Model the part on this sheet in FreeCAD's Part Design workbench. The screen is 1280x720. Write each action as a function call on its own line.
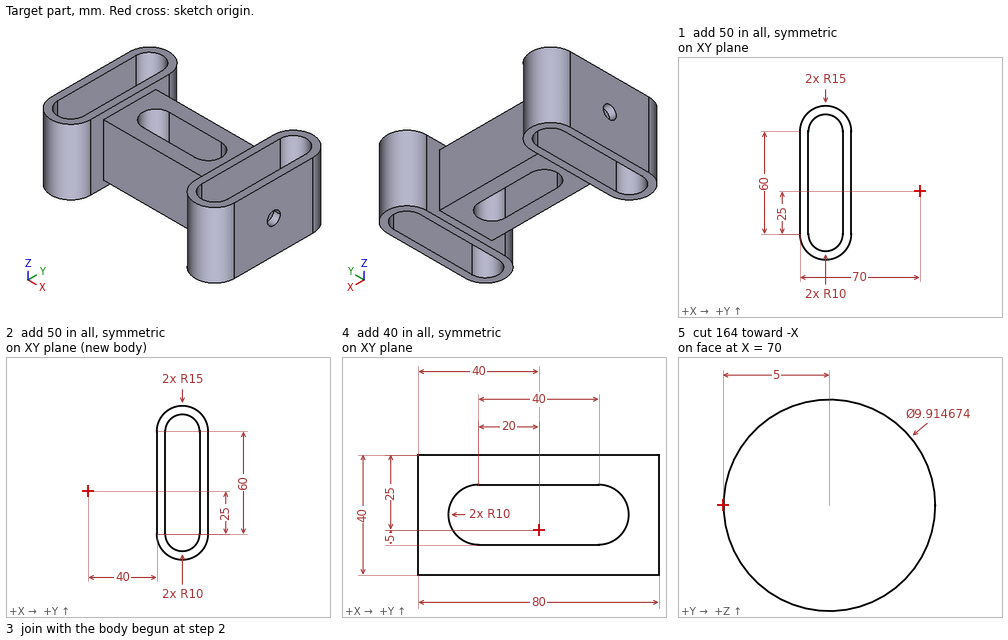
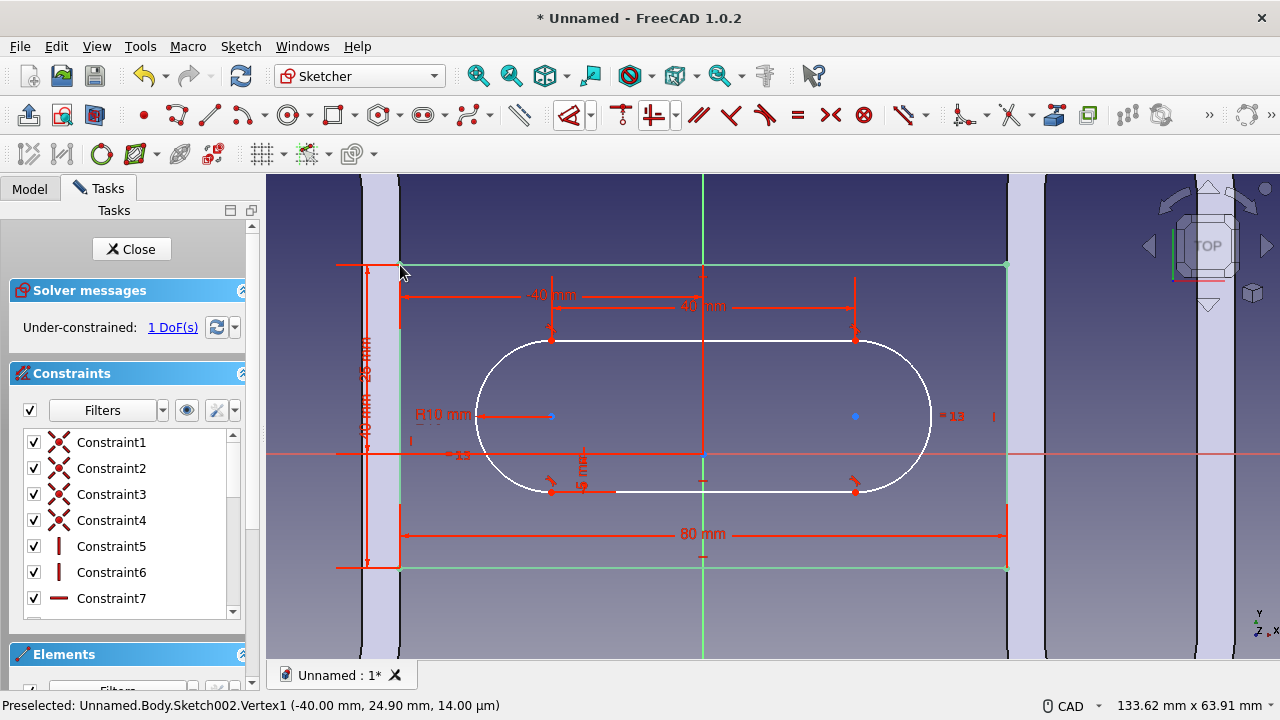
click(552, 341)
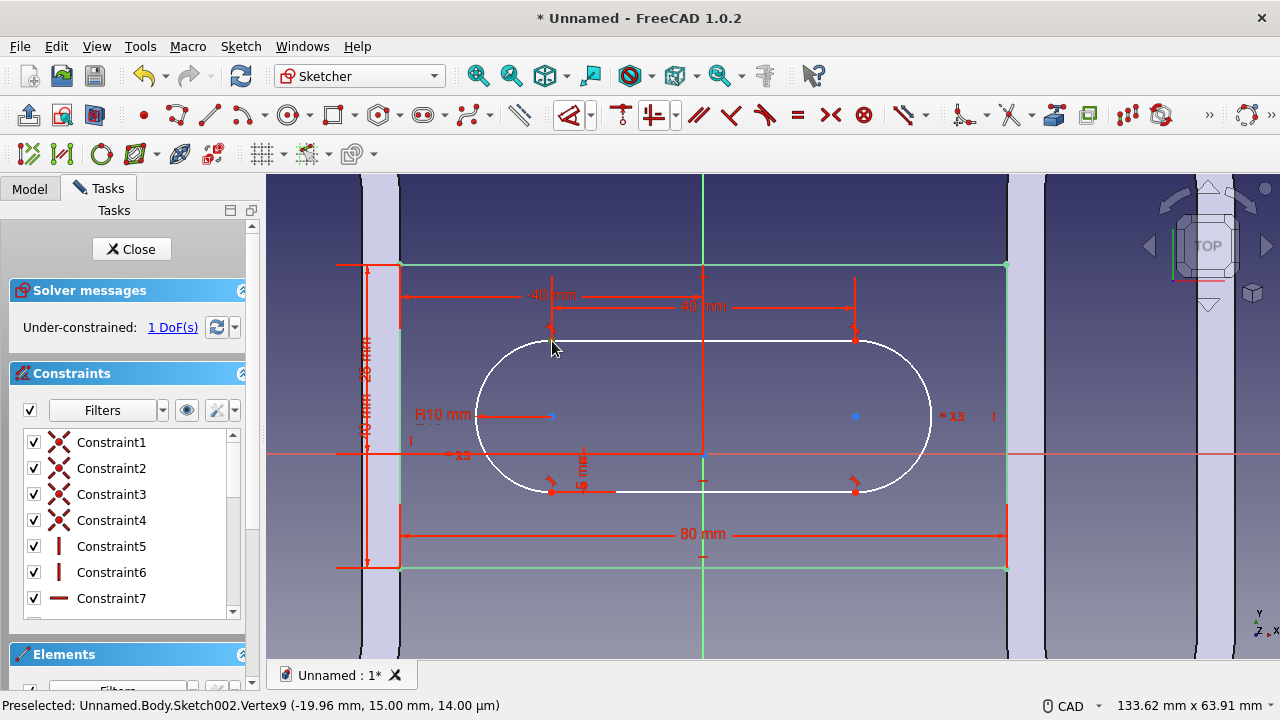
click(590, 116)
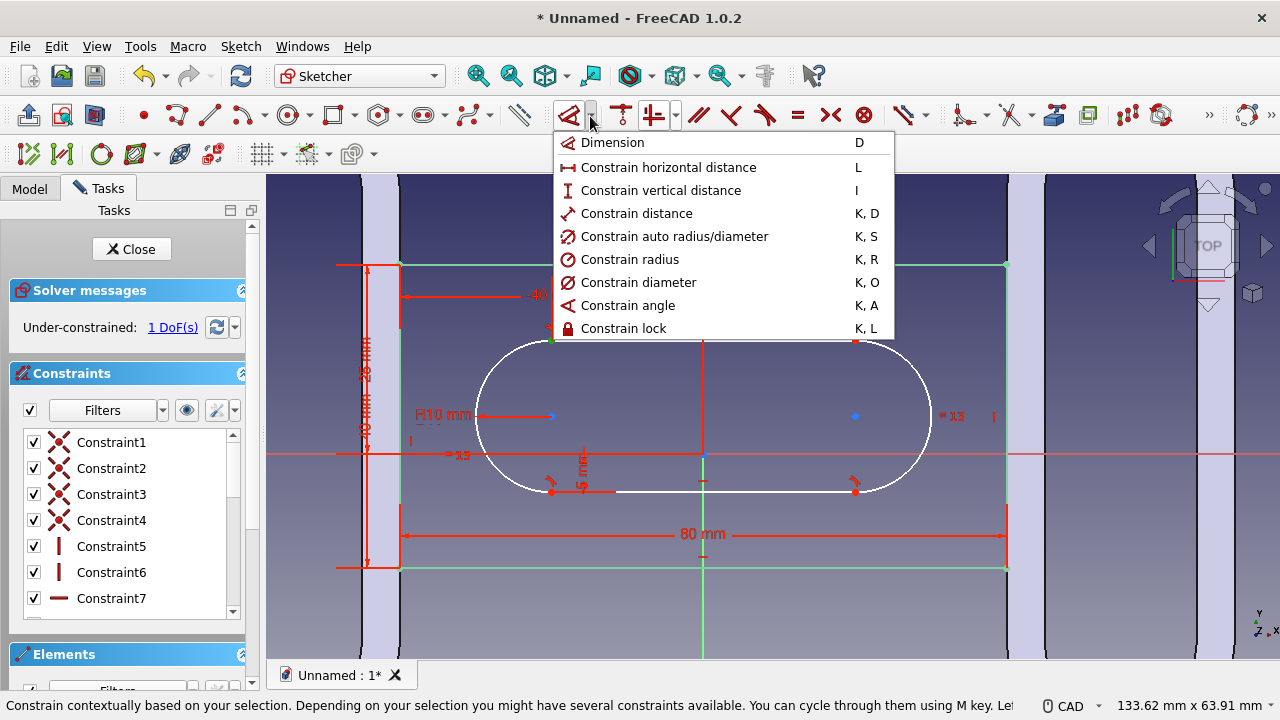
click(724, 168)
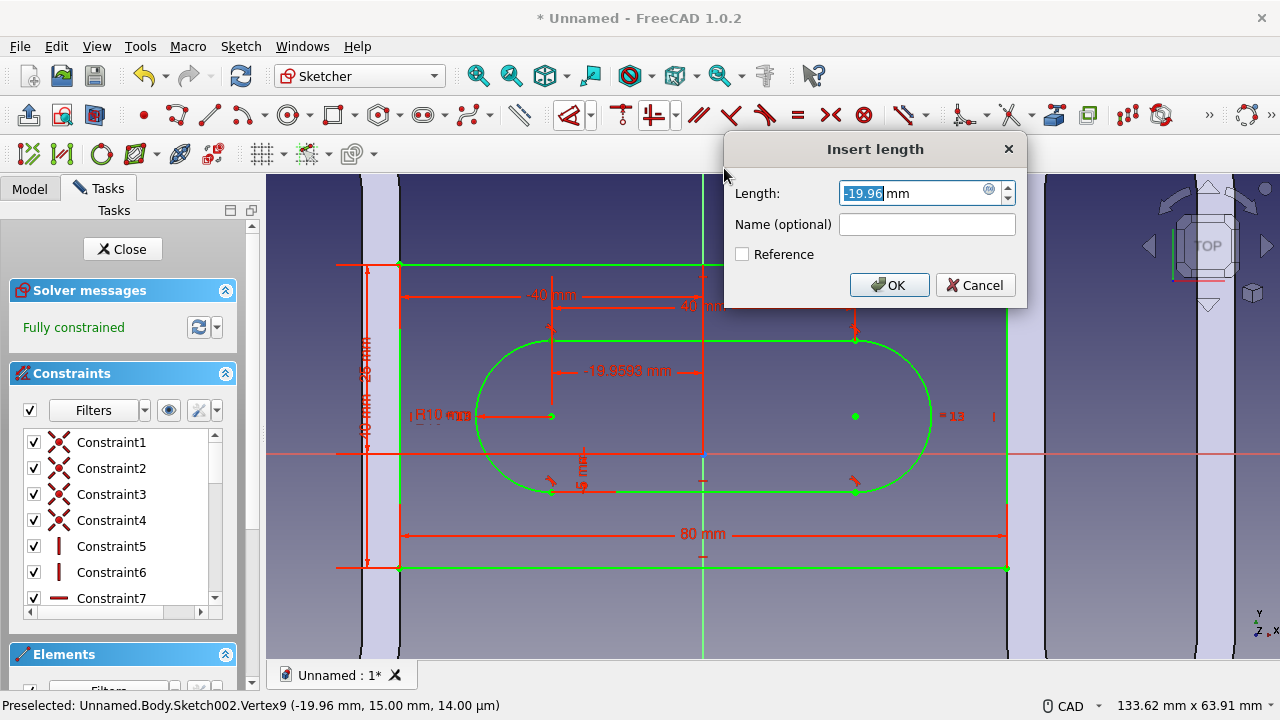
text(-20)
key(Return)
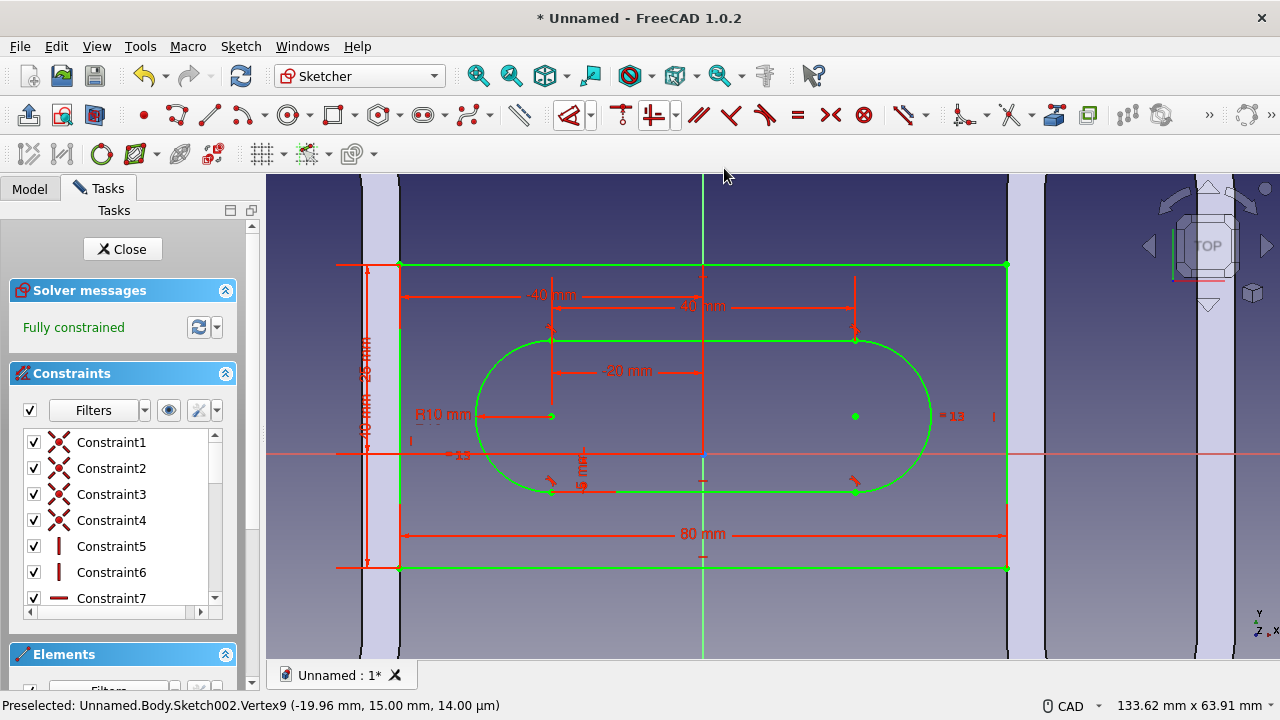
click(123, 249)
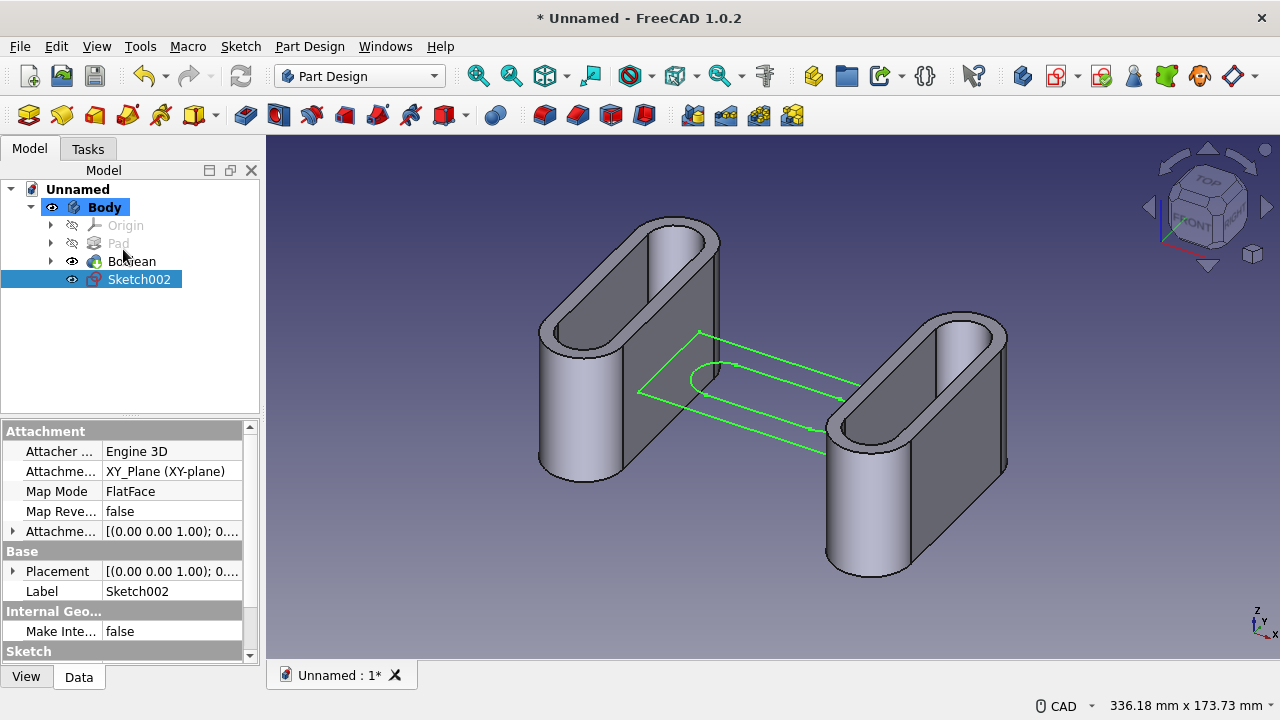
click(29, 116)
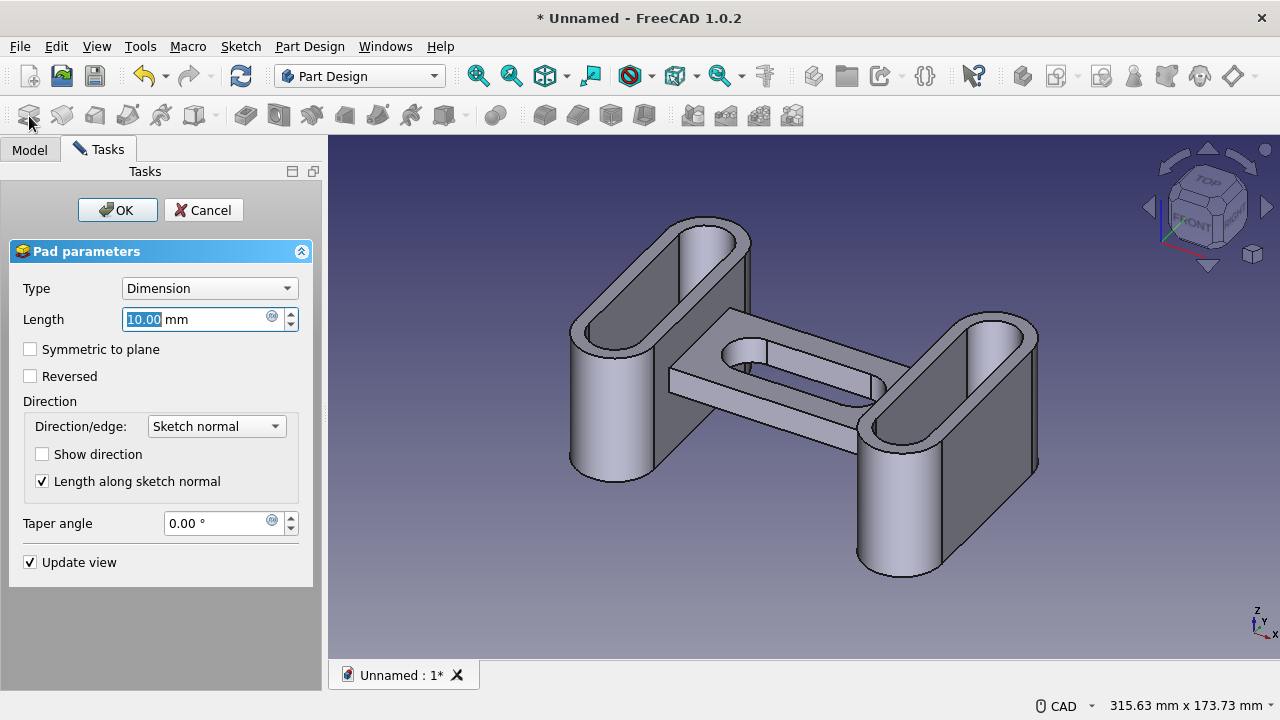
text(40)
key(Tab)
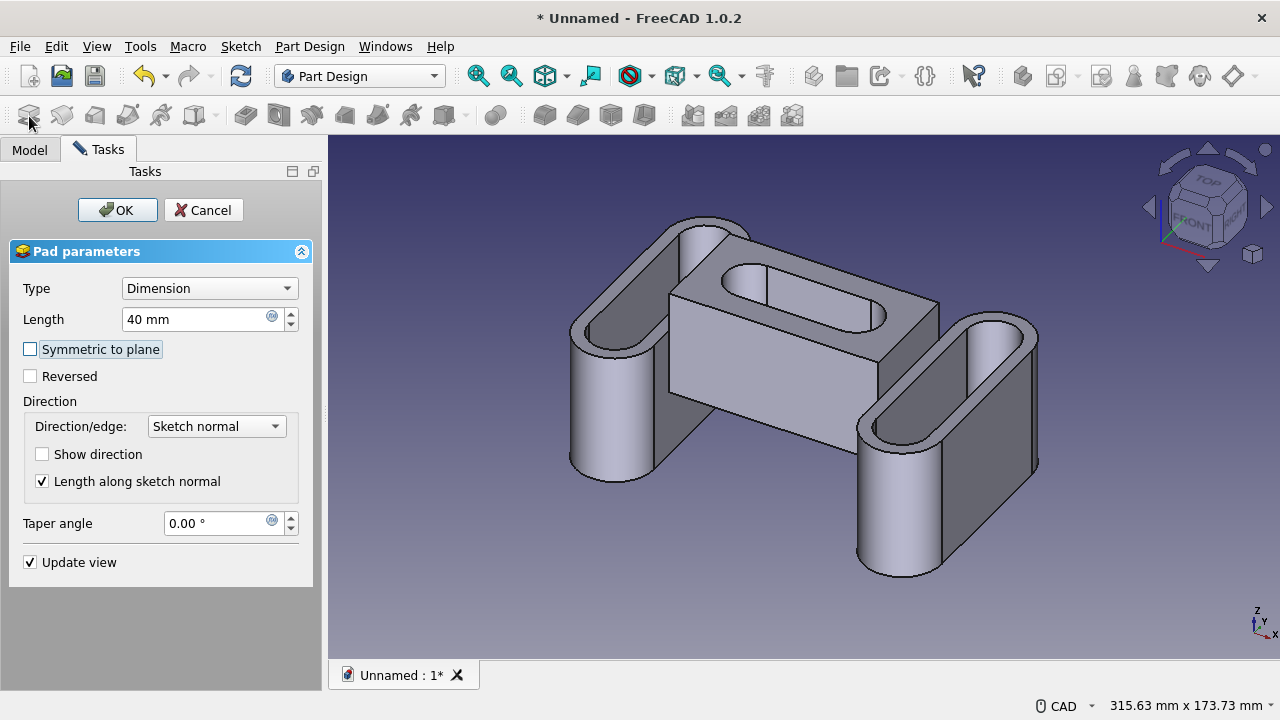
click(31, 349)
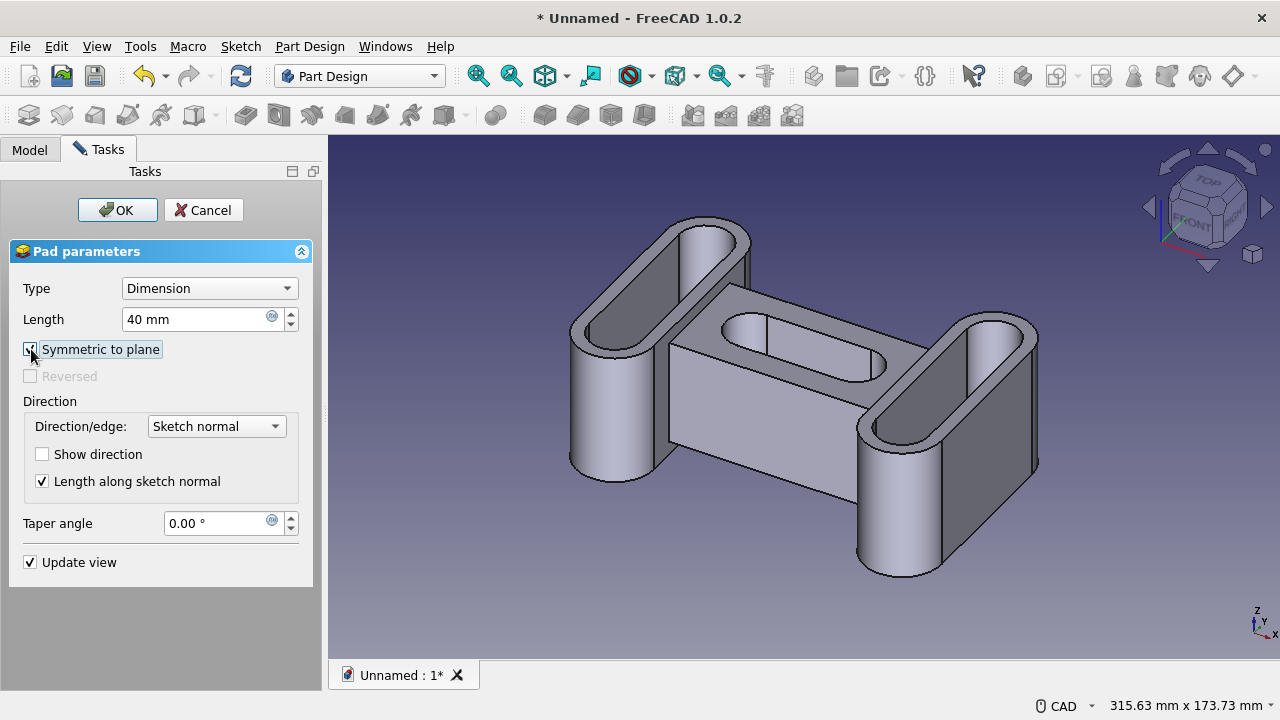
click(118, 210)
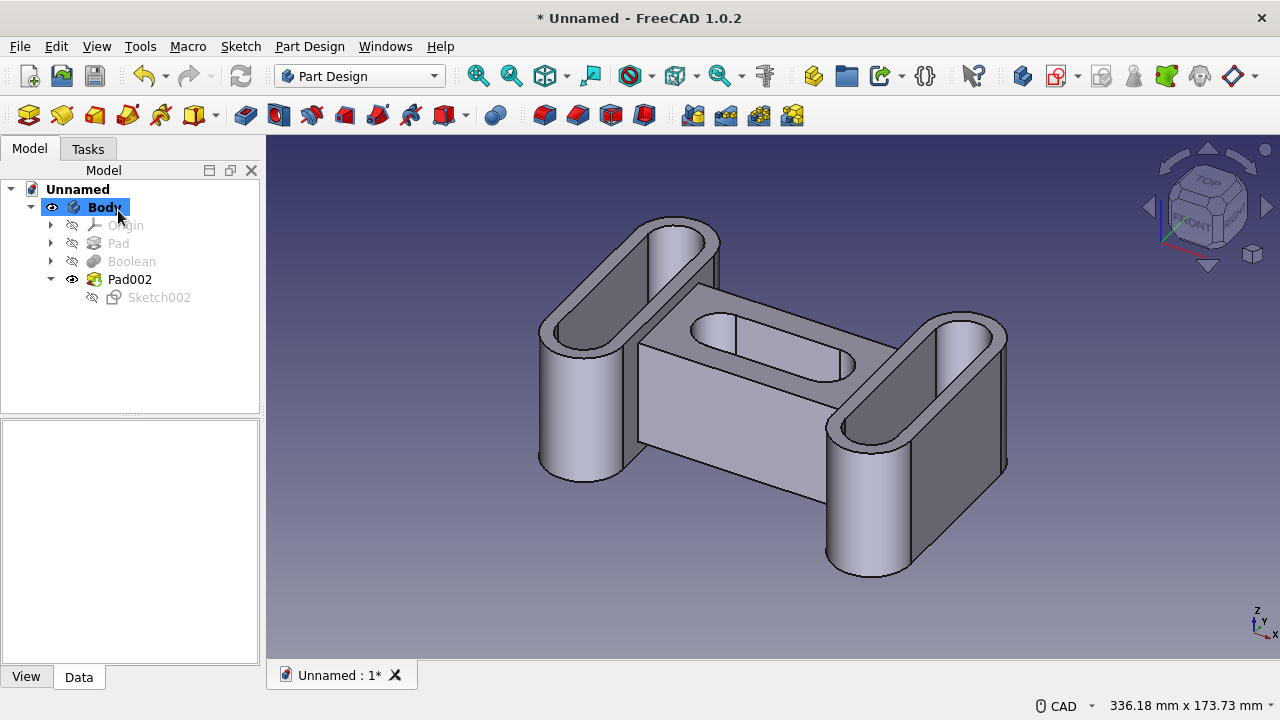
click(956, 457)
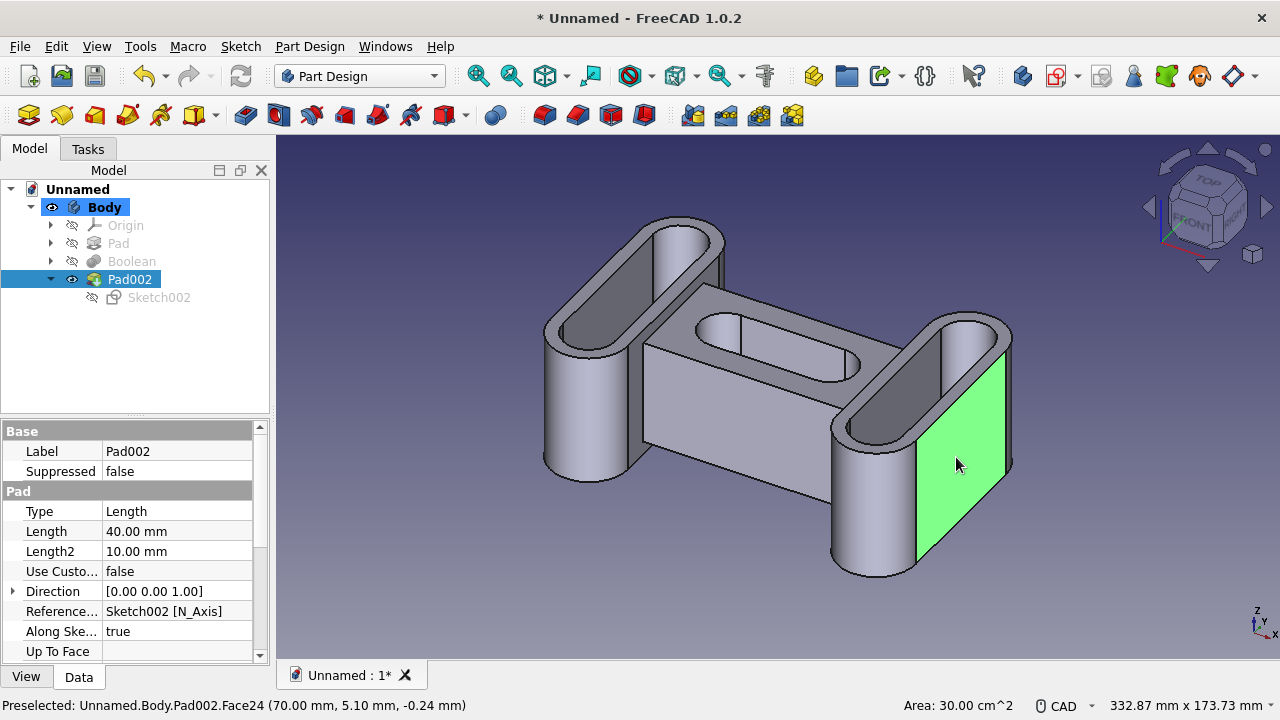
click(1056, 76)